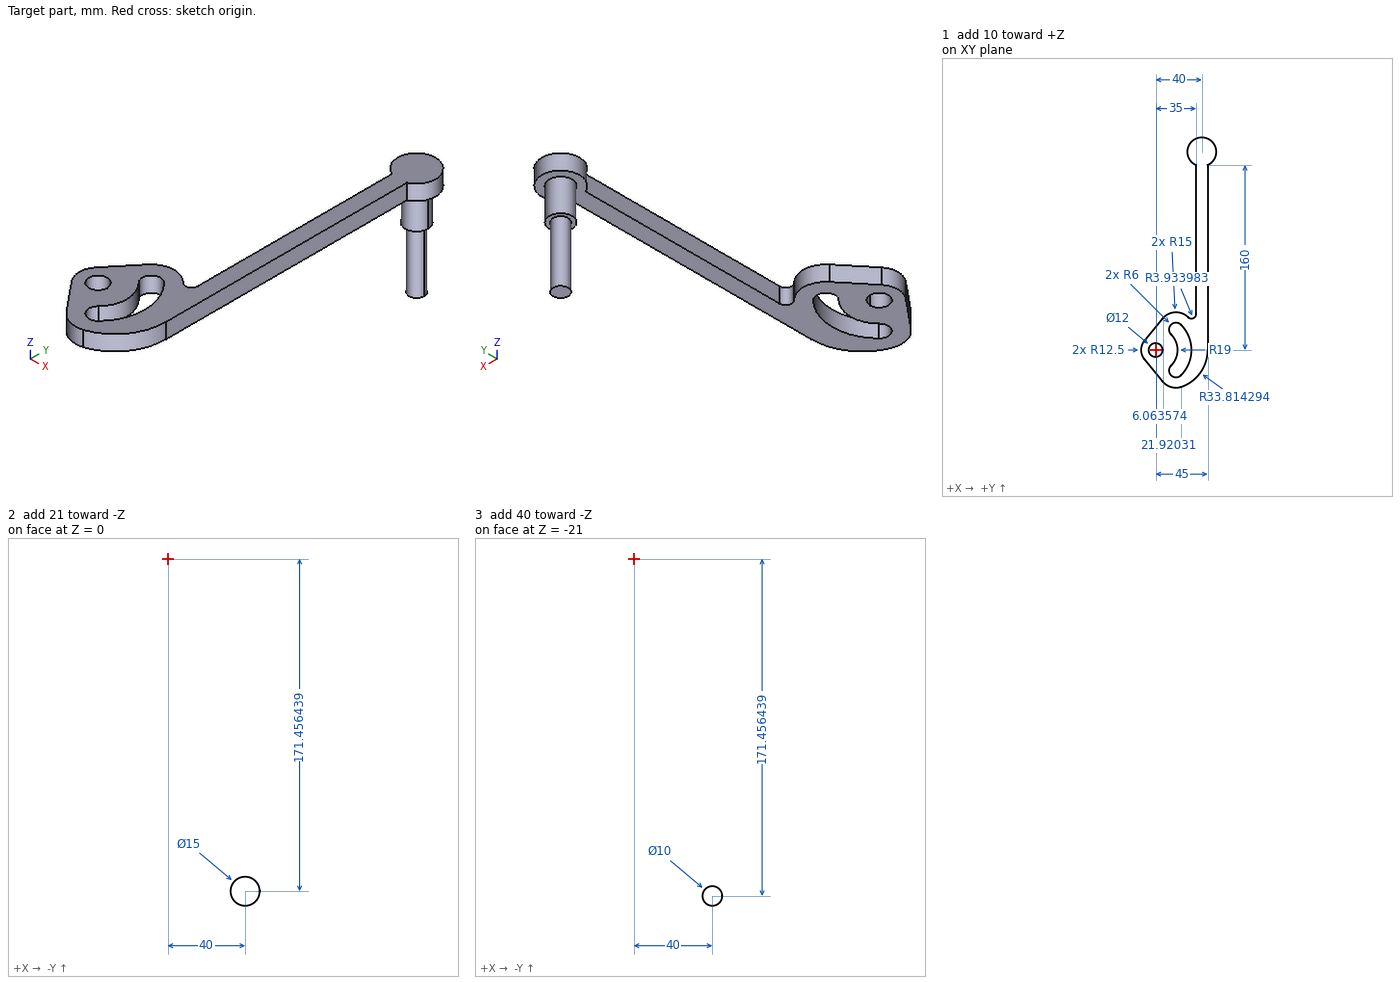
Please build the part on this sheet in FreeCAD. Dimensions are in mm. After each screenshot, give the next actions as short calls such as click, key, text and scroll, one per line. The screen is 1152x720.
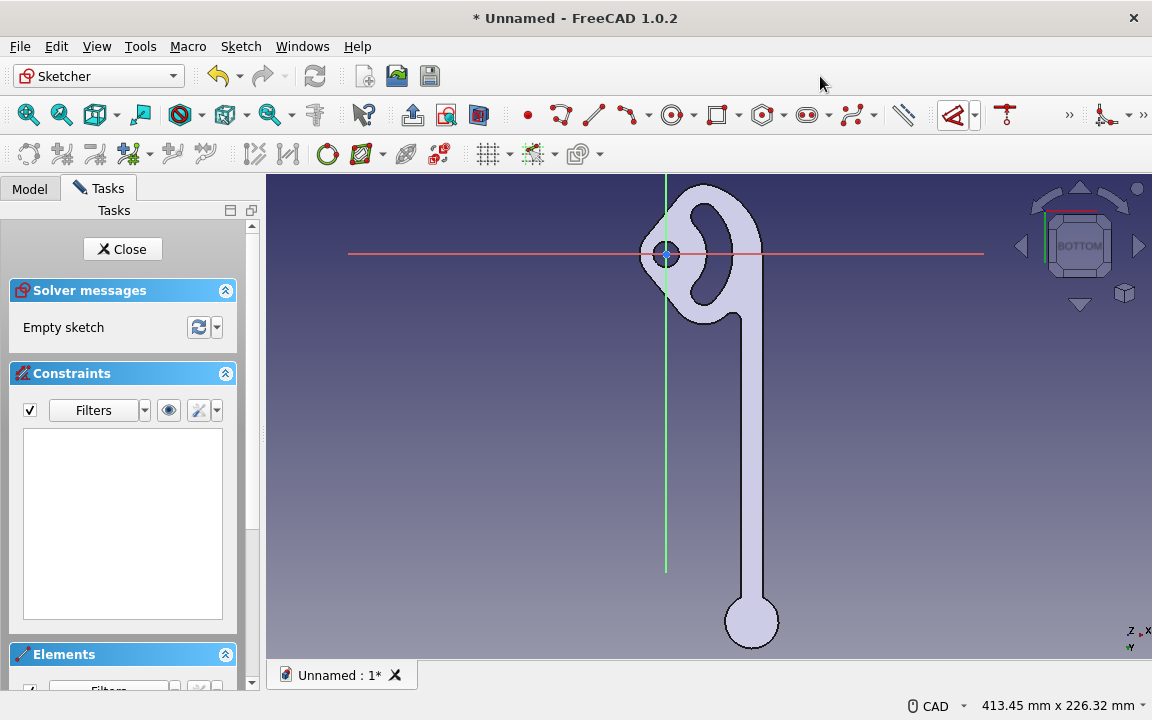
scroll(640, 416, down, 5)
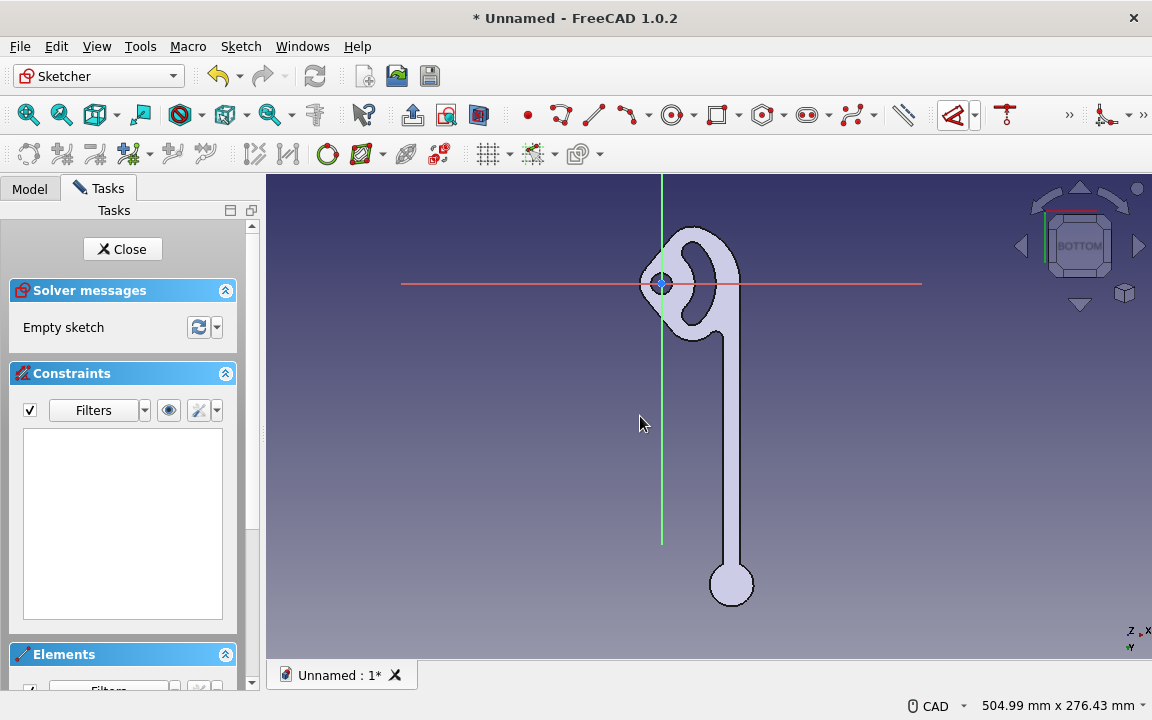
scroll(684, 496, up, 15)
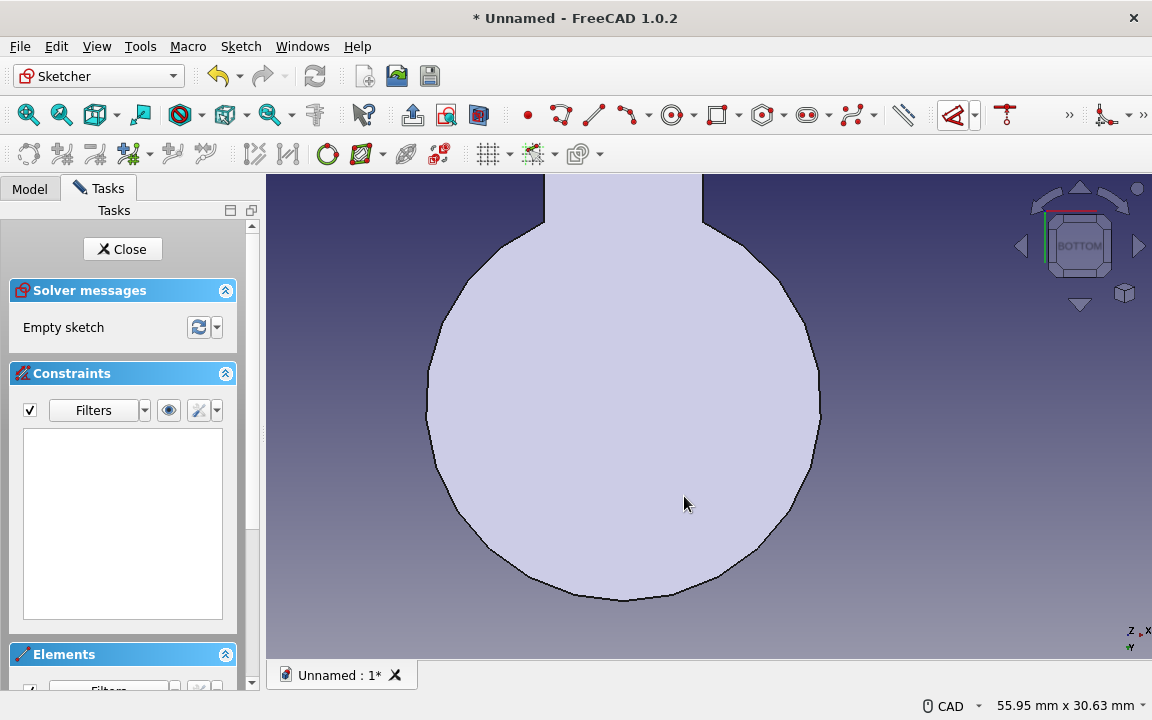
key(g)
key(c)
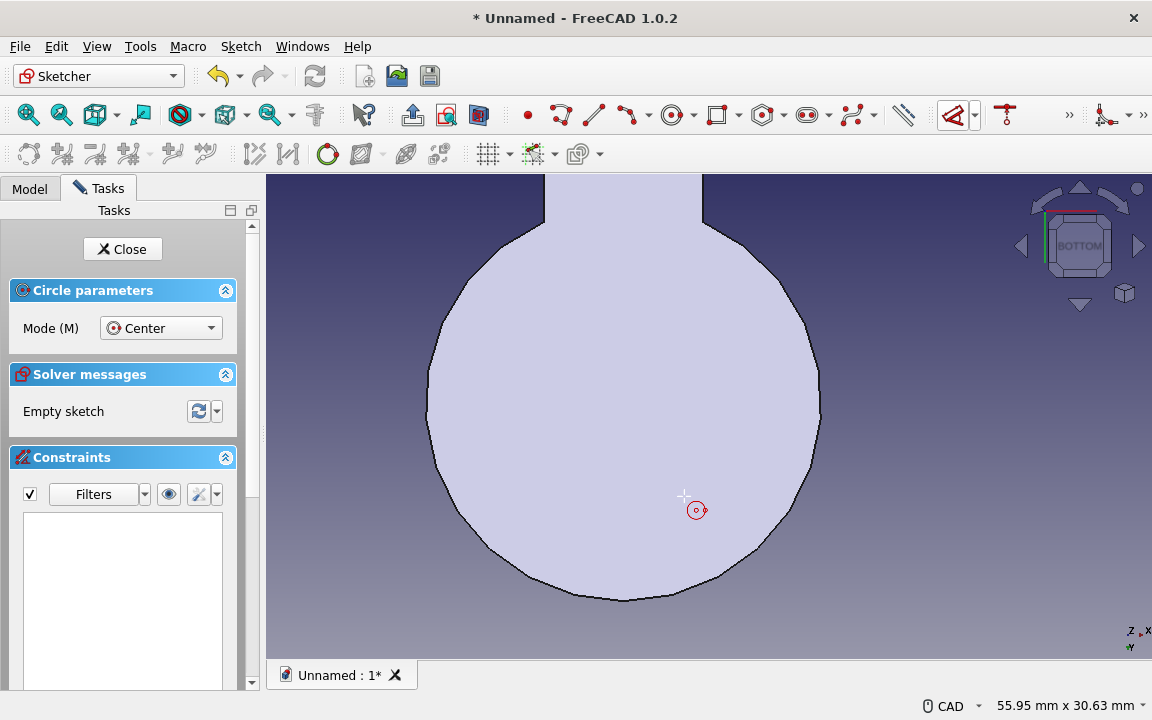
click(623, 403)
click(707, 319)
key(Escape)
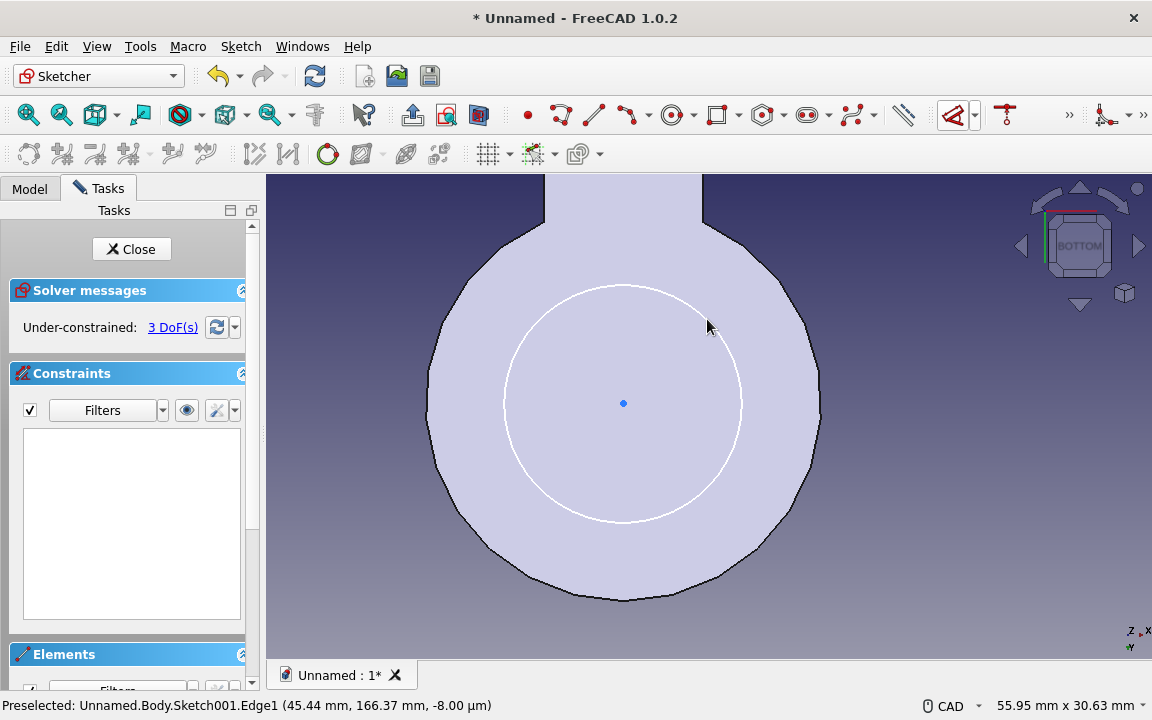
key(d)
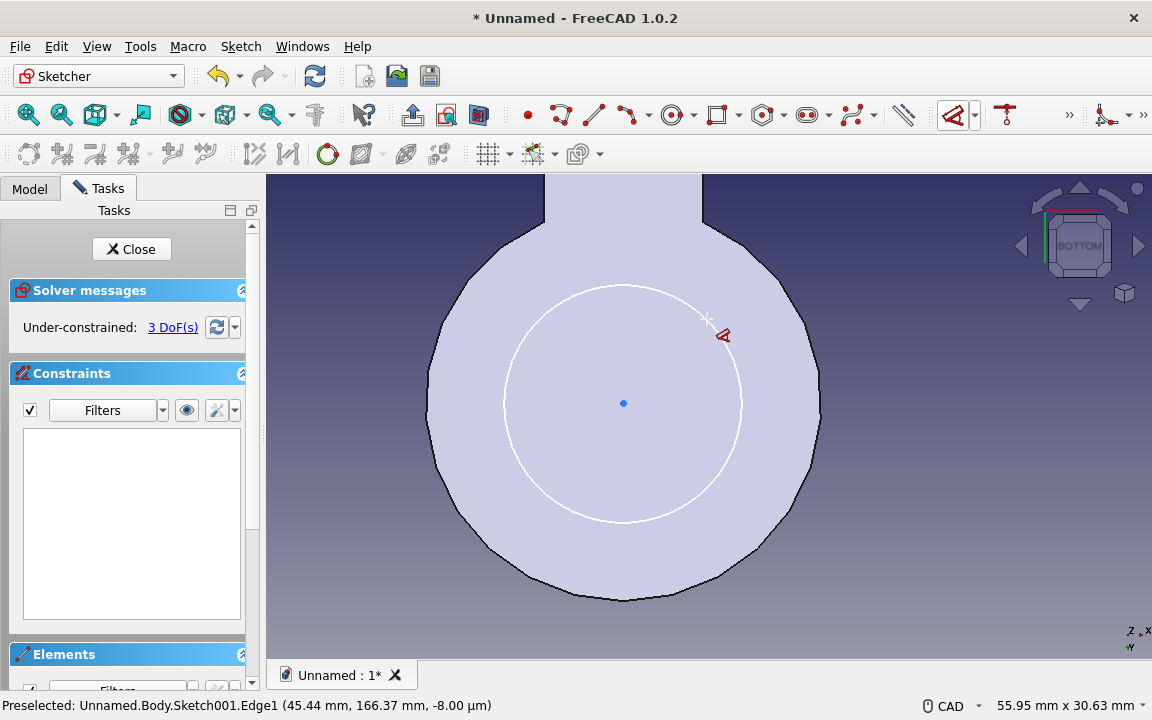
click(707, 320)
click(730, 297)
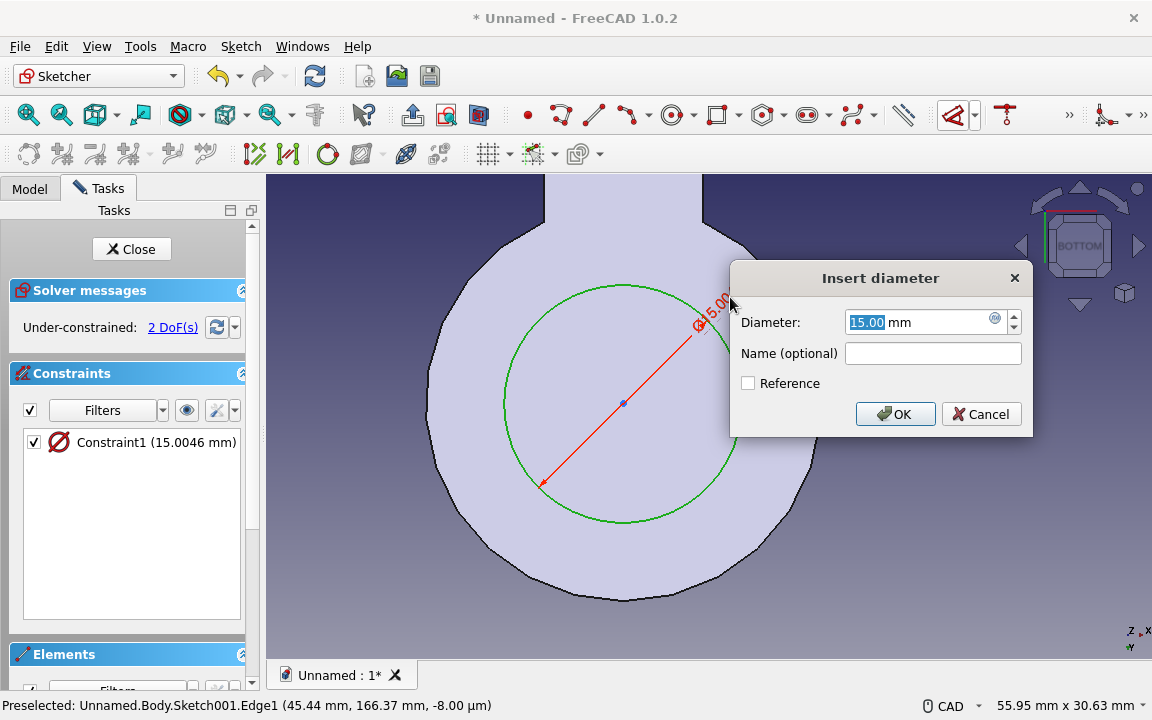
text(15)
key(Return)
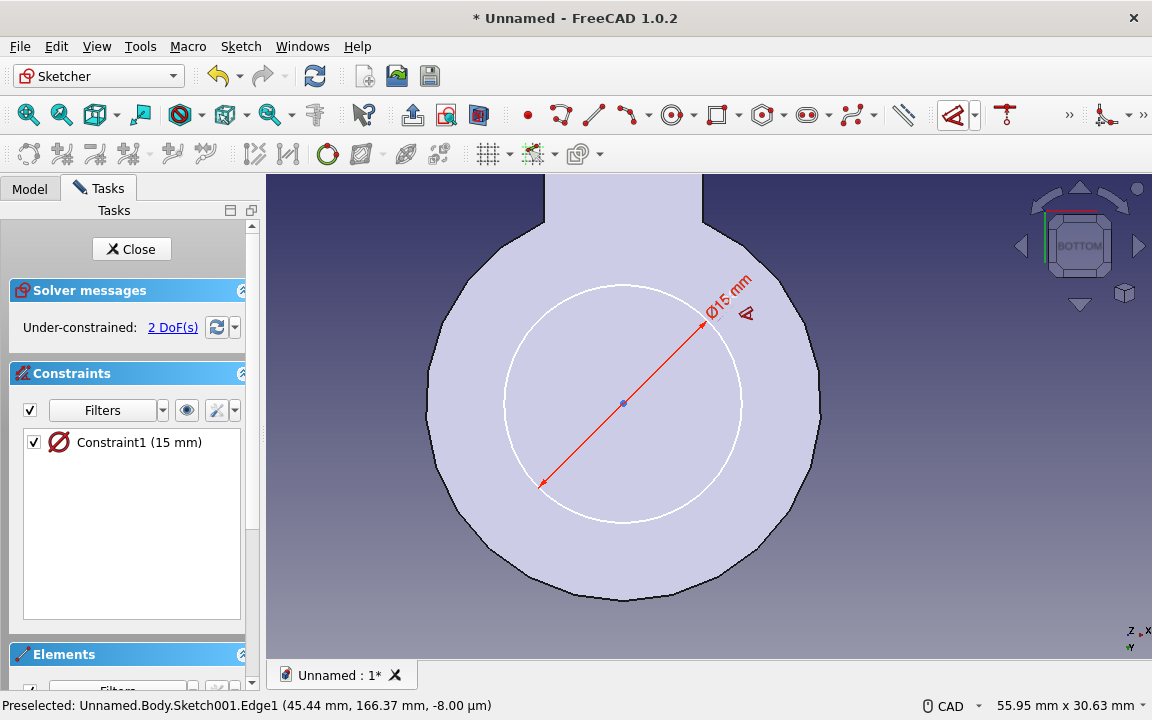
click(623, 404)
click(459, 438)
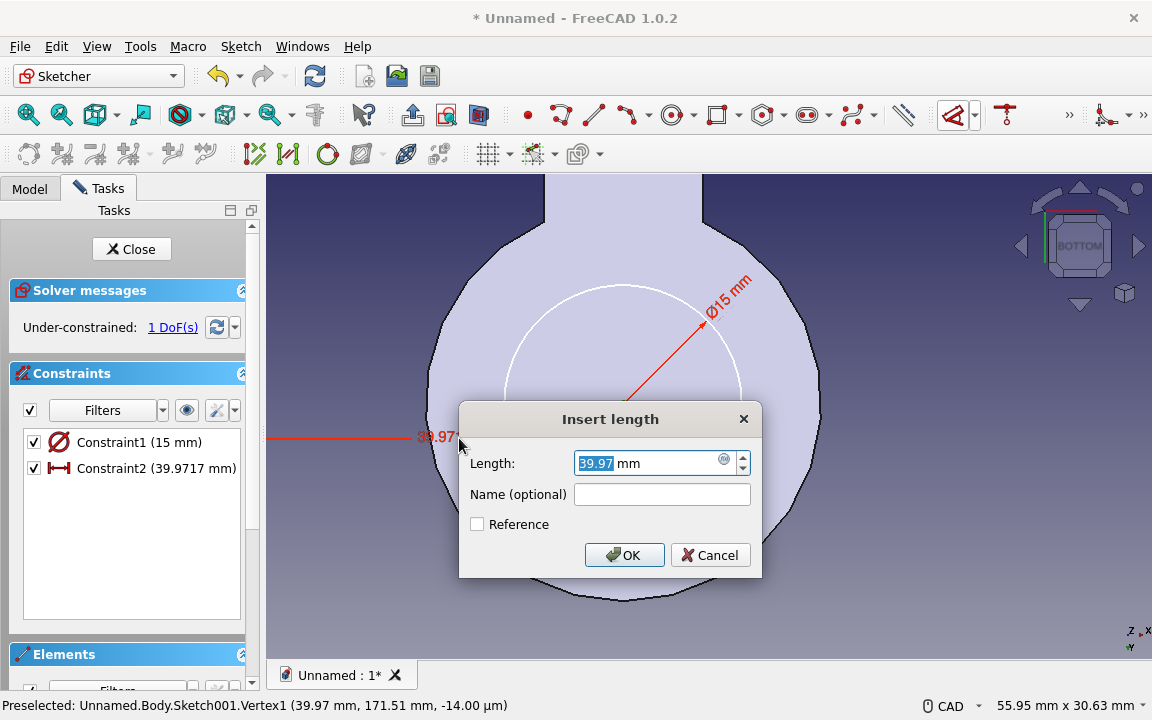
text(40)
key(Return)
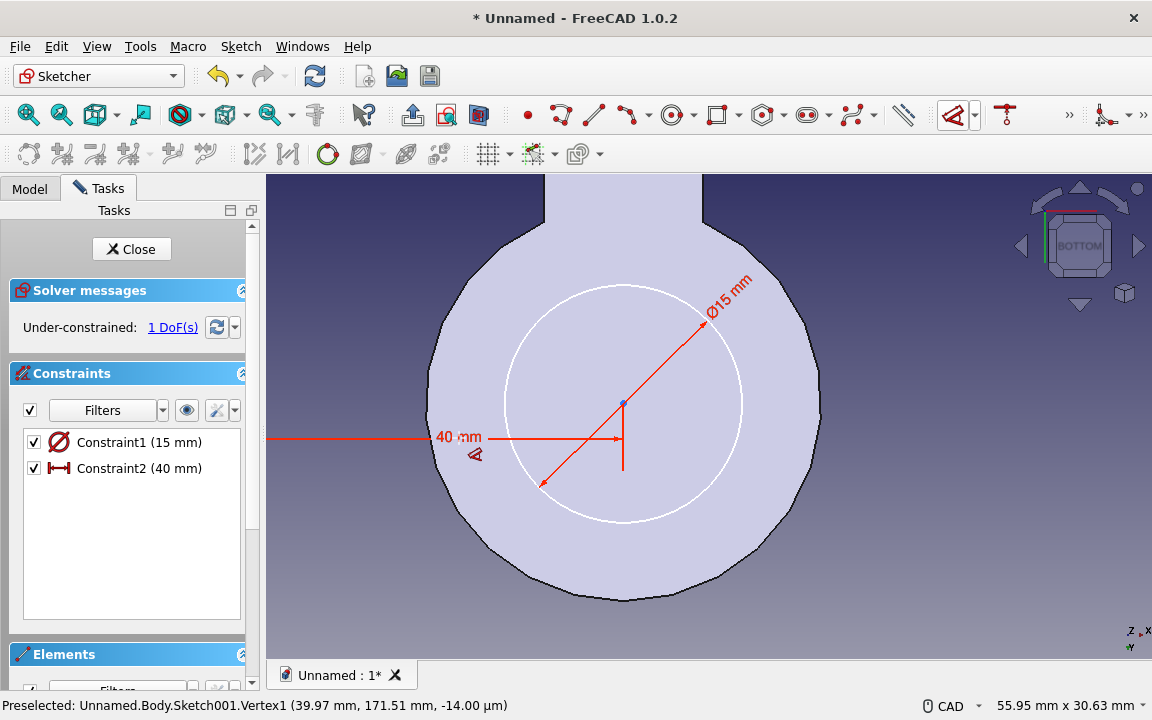
click(623, 404)
click(657, 257)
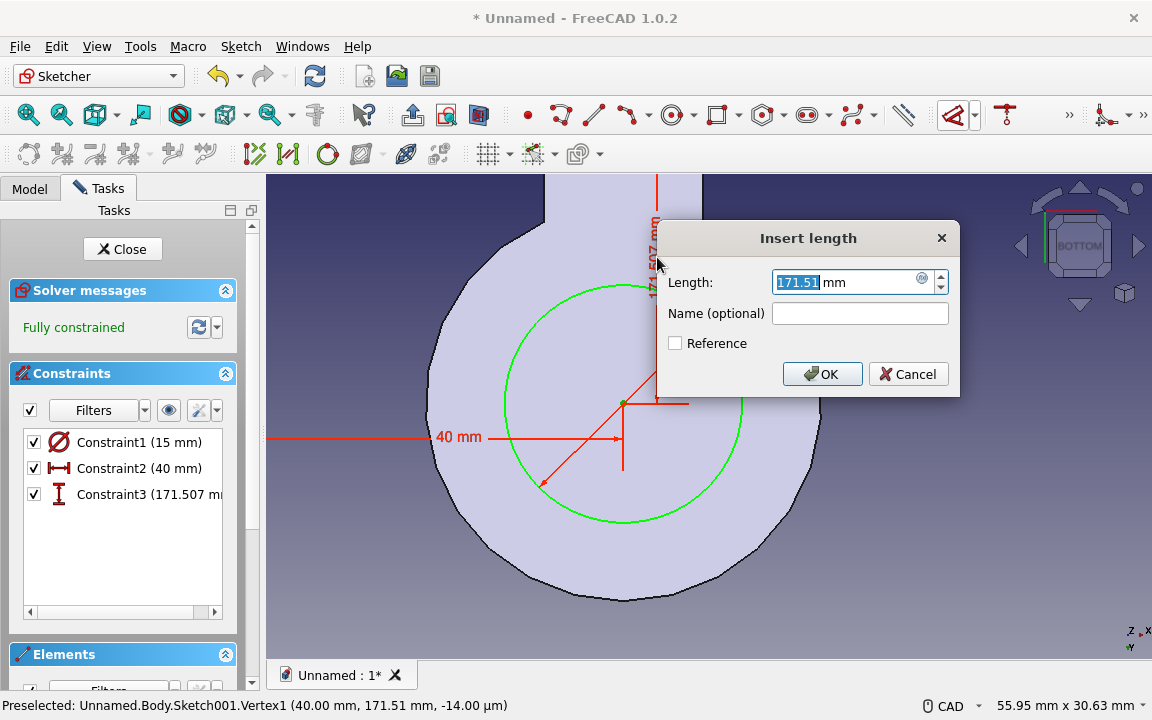
text(171.456439)
key(Return)
key(Escape)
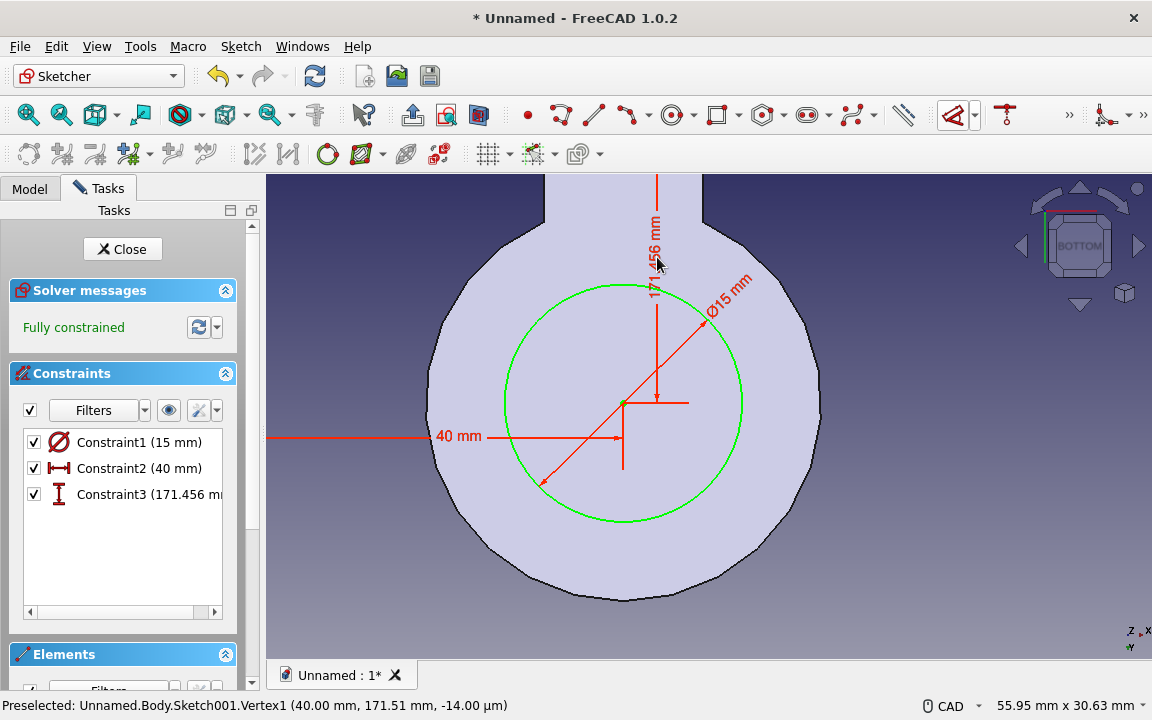
click(123, 249)